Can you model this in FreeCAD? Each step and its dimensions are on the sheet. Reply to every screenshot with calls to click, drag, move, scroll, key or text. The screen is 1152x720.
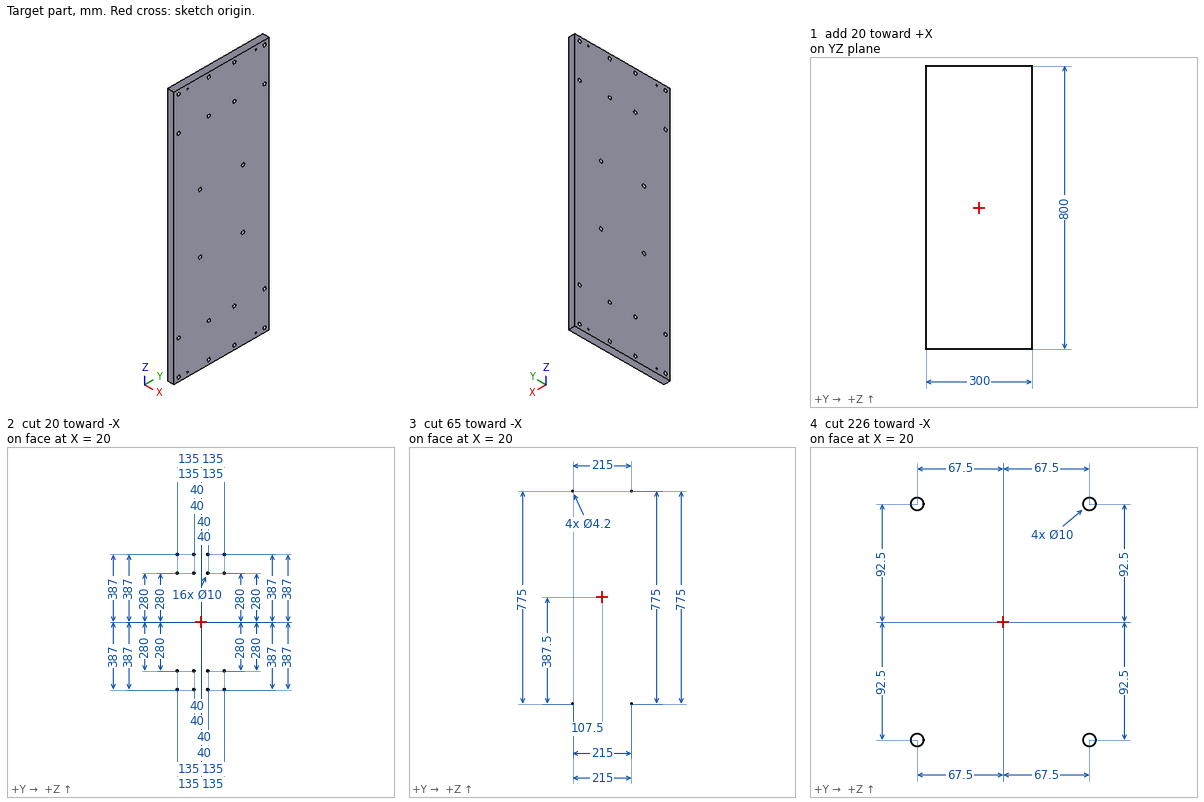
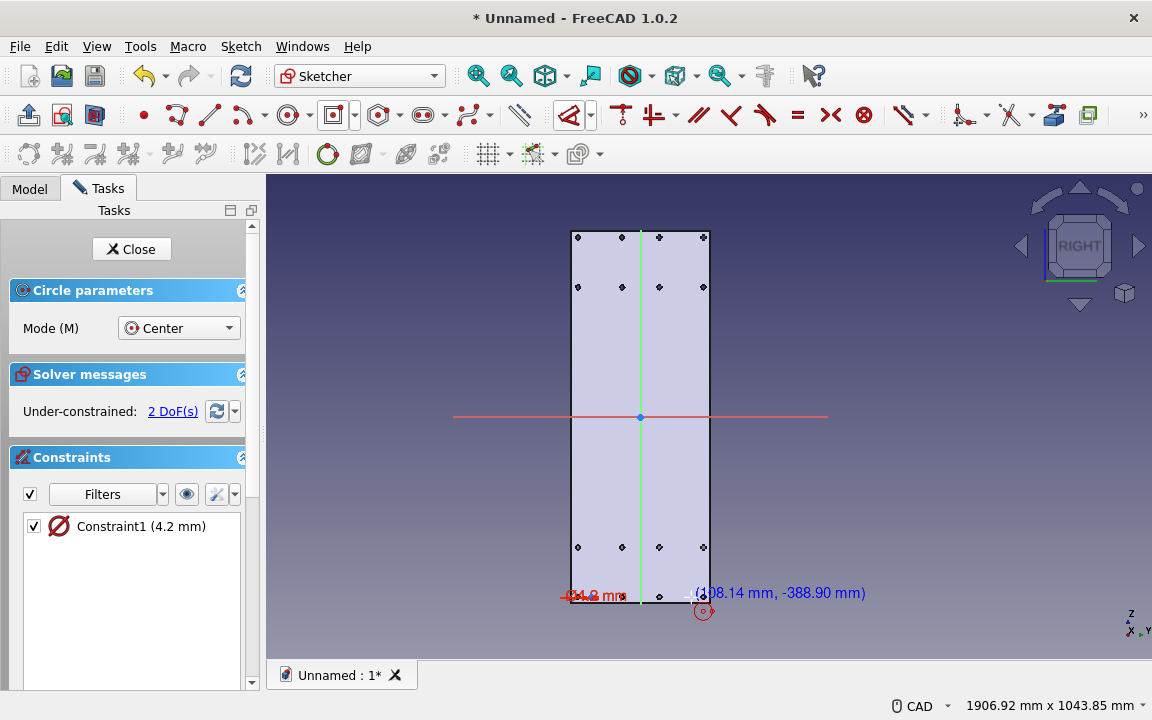
click(691, 597)
move(691, 597)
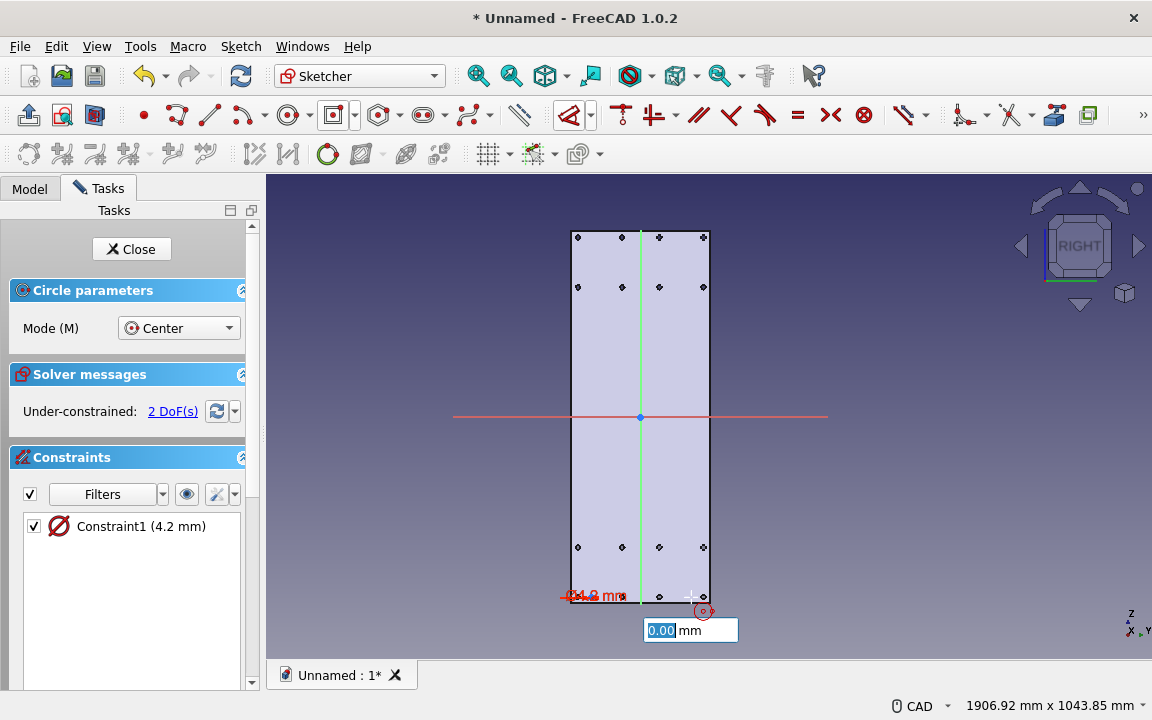
text(4.2)
key(Return)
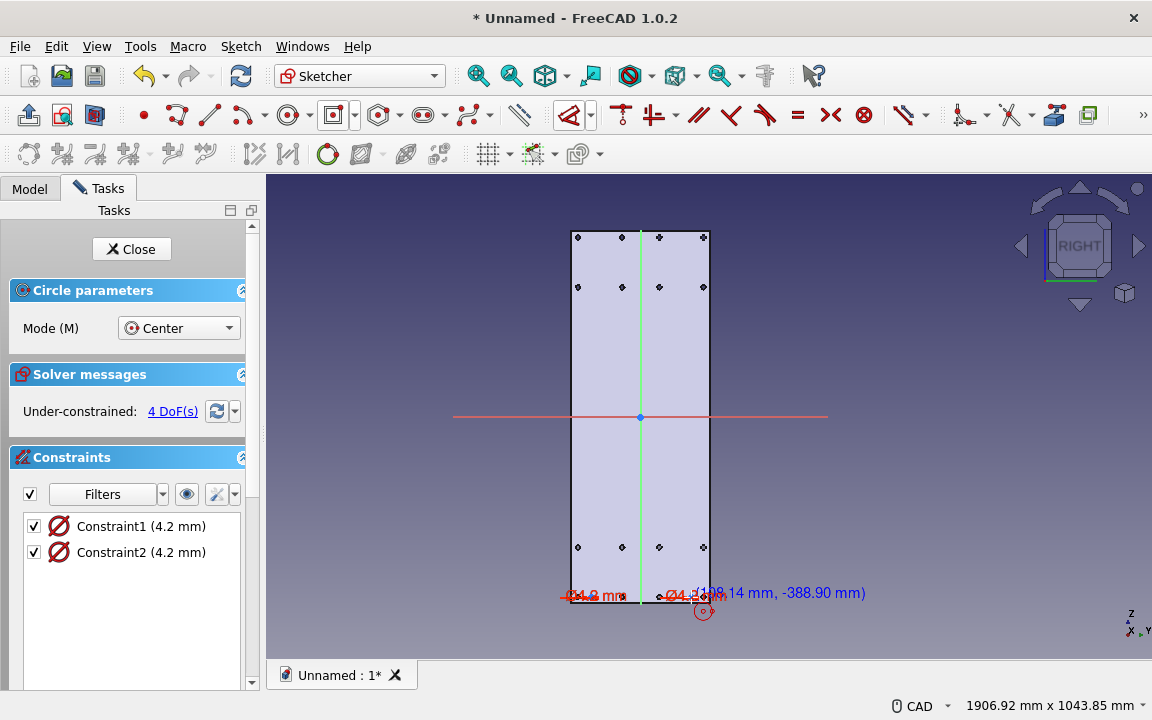
scroll(591, 237, up, 16)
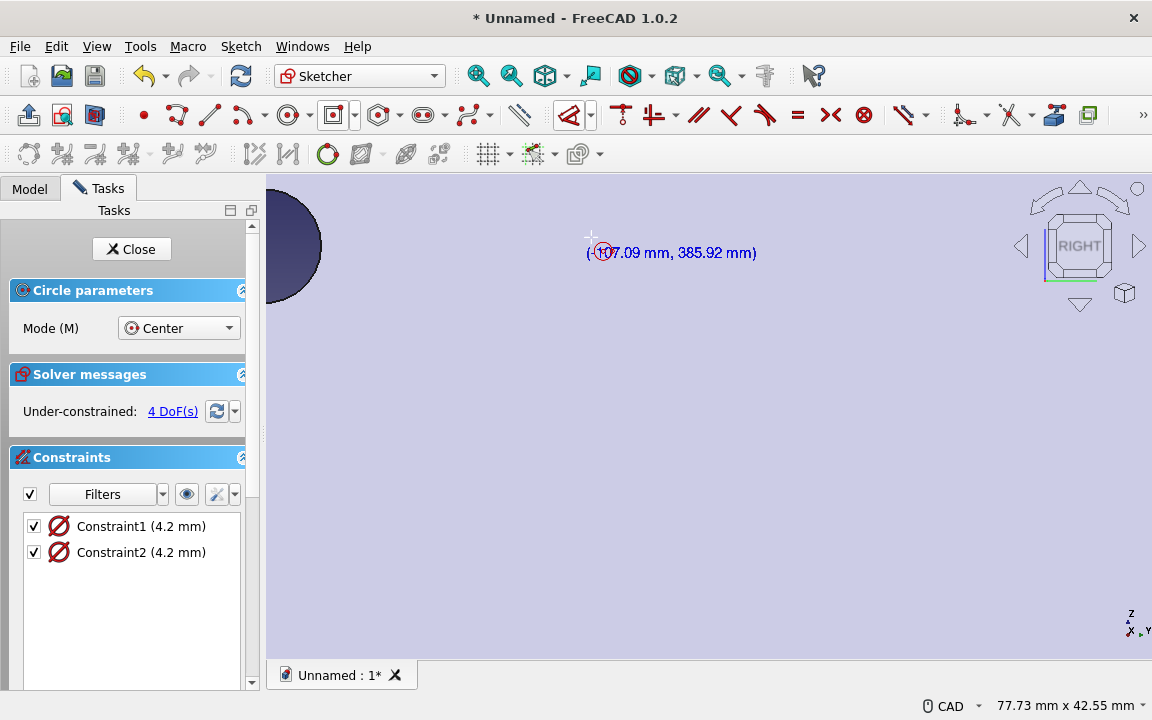
scroll(591, 236, down, 16)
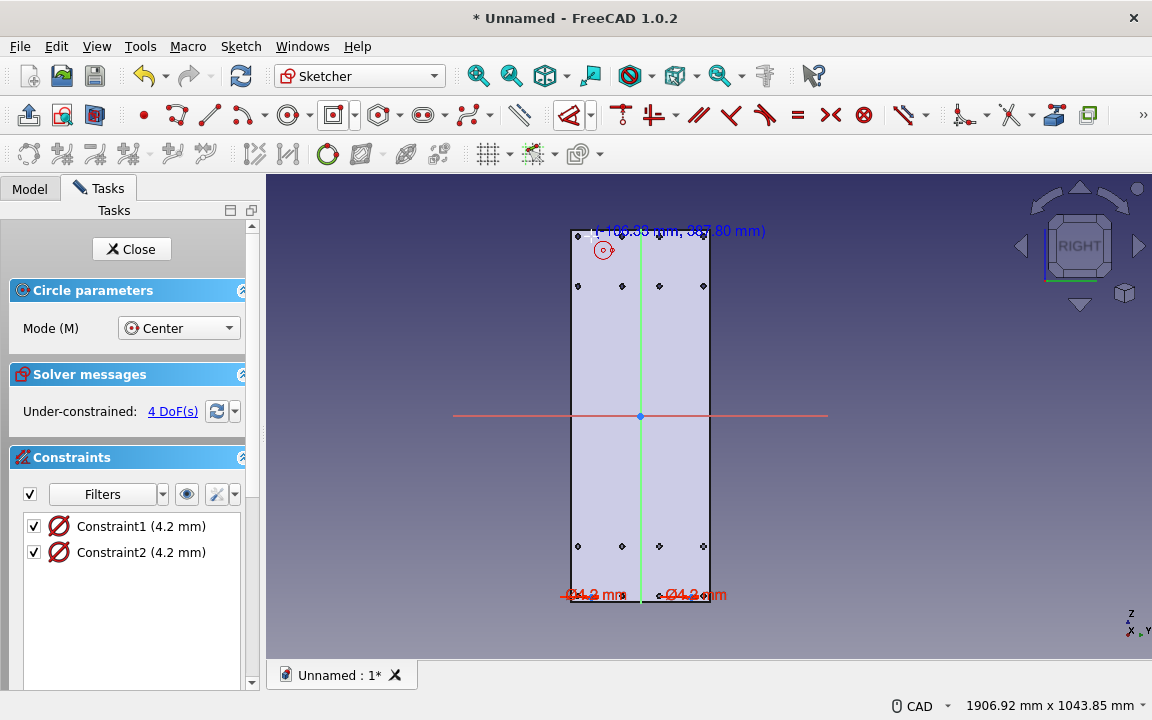
click(591, 236)
move(592, 236)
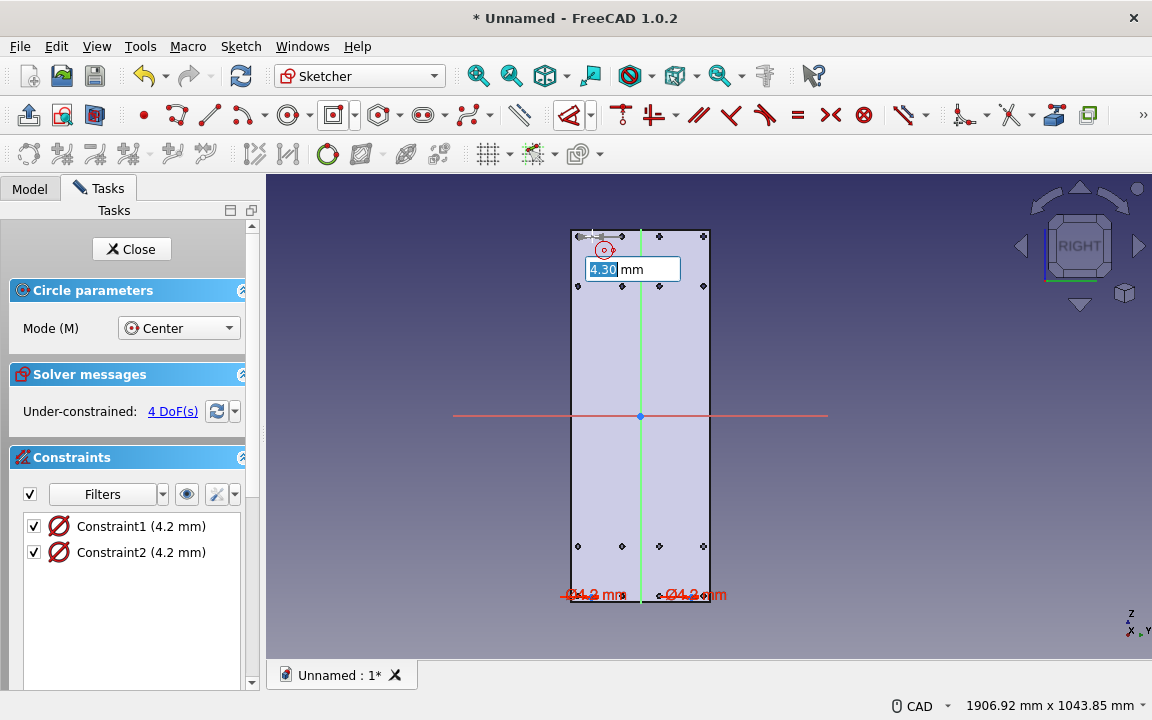
text(4.2)
key(Return)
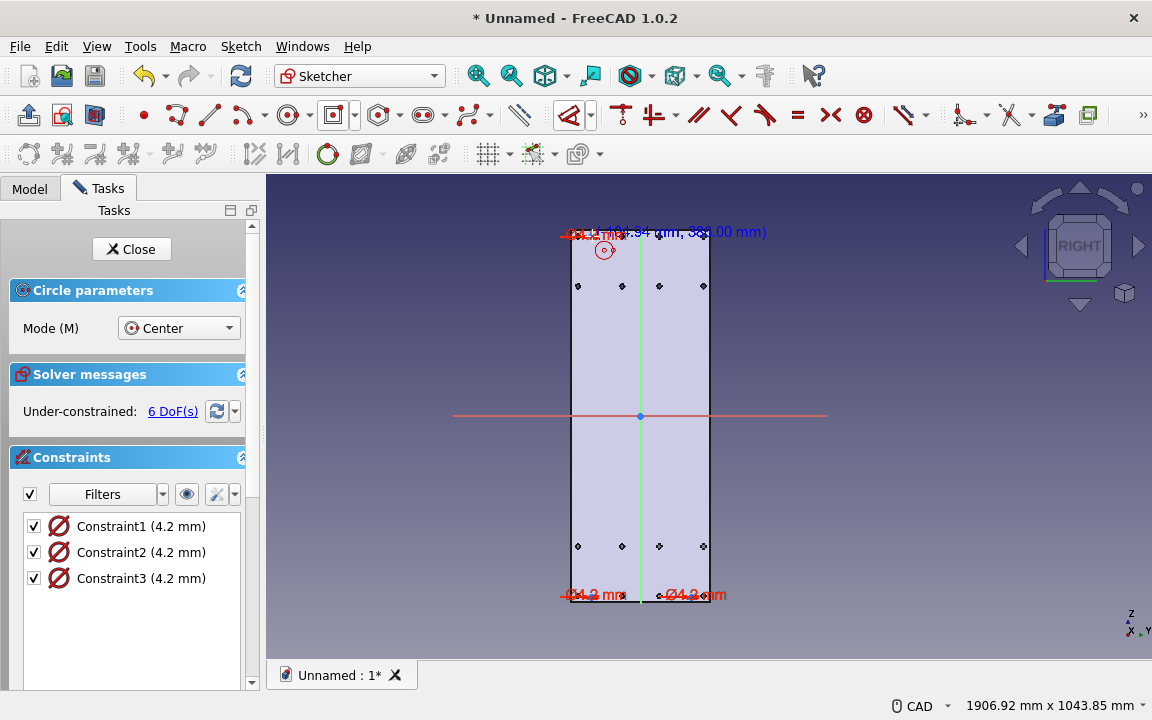
scroll(691, 236, up, 16)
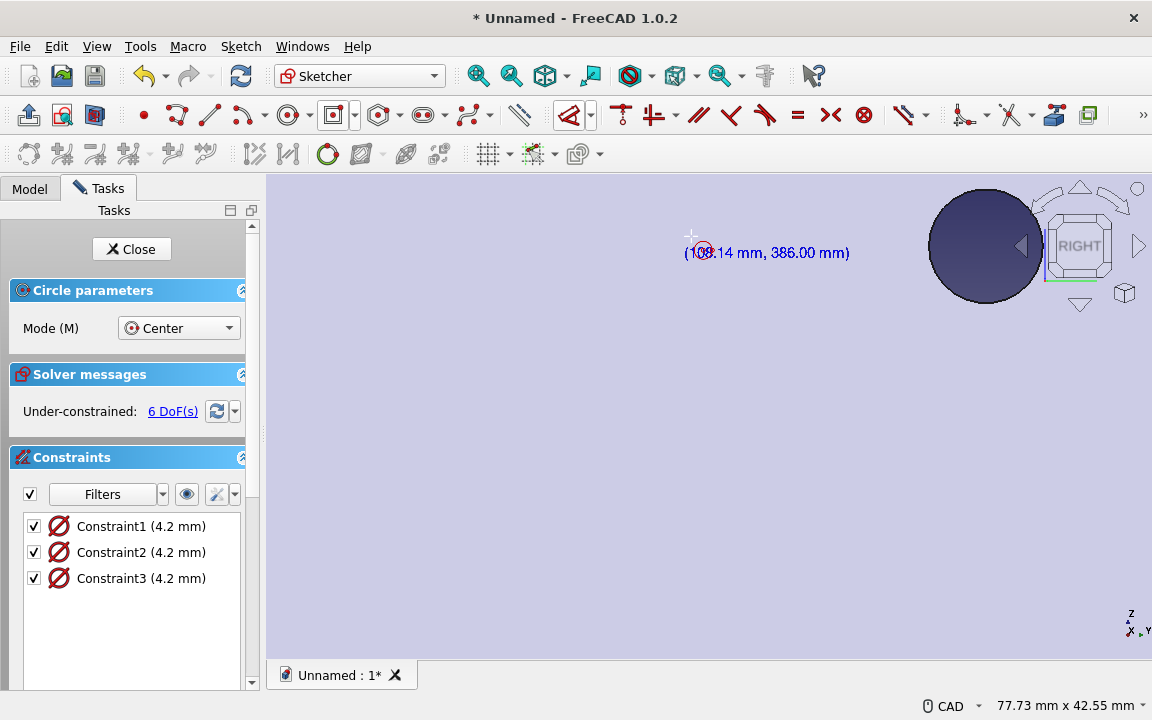
scroll(691, 236, down, 16)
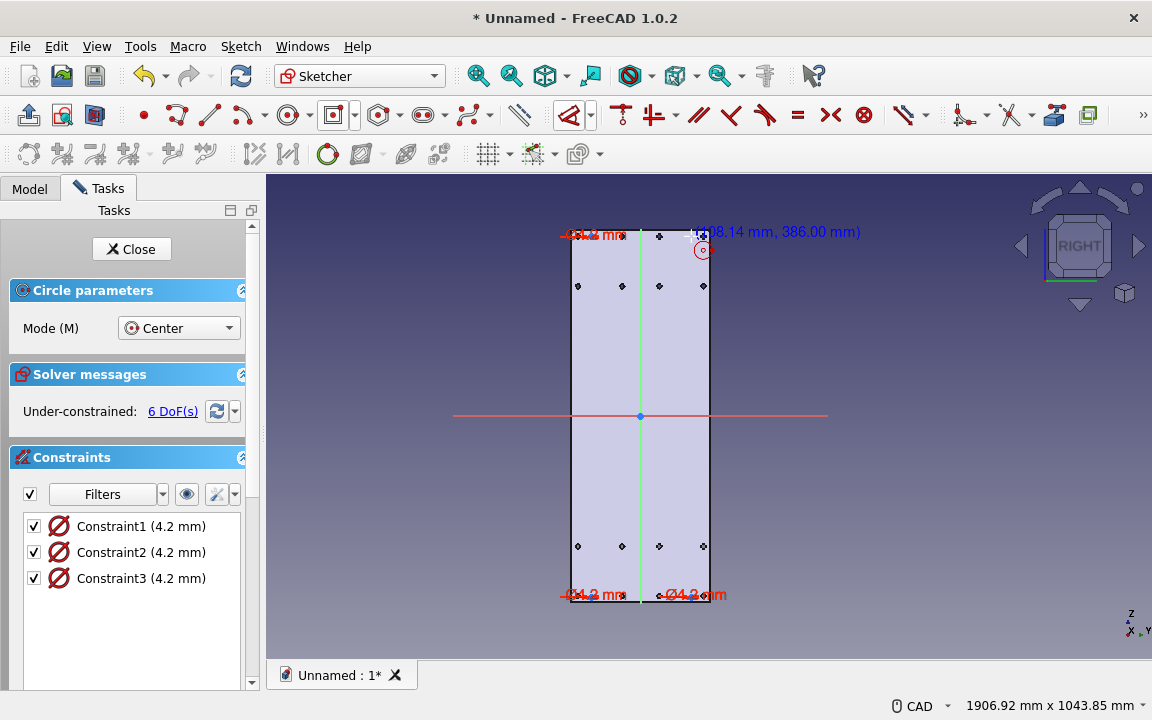
click(691, 236)
move(691, 236)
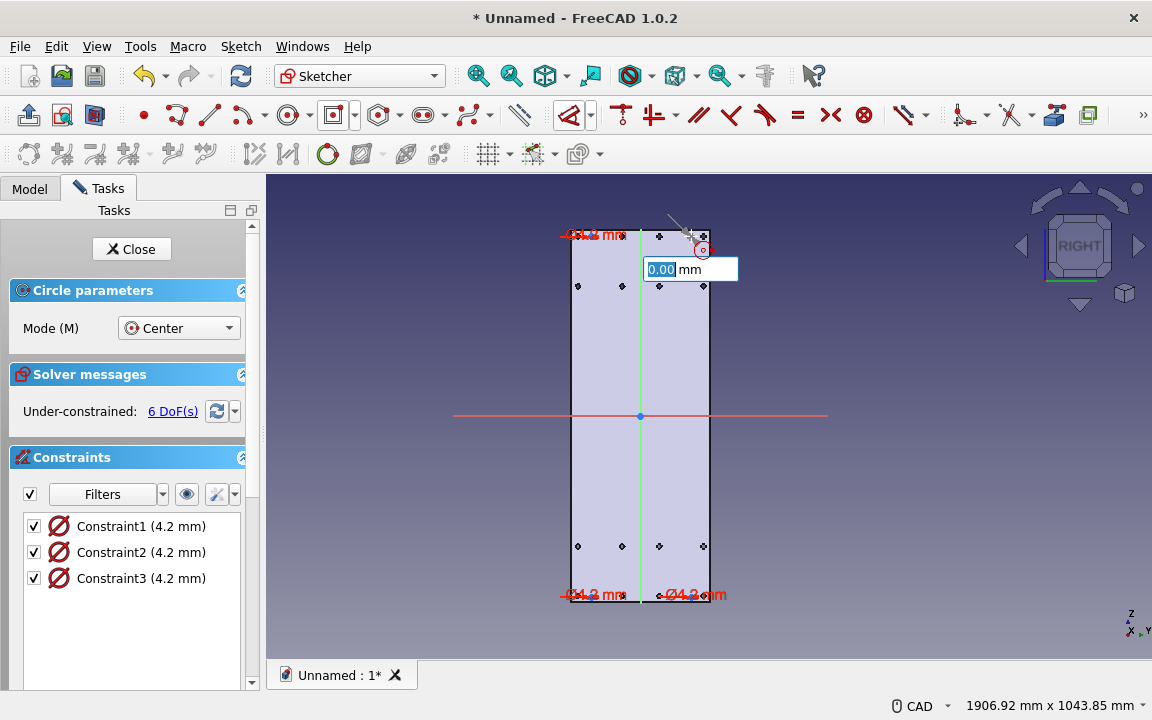
text(4.2)
key(Return)
key(Escape)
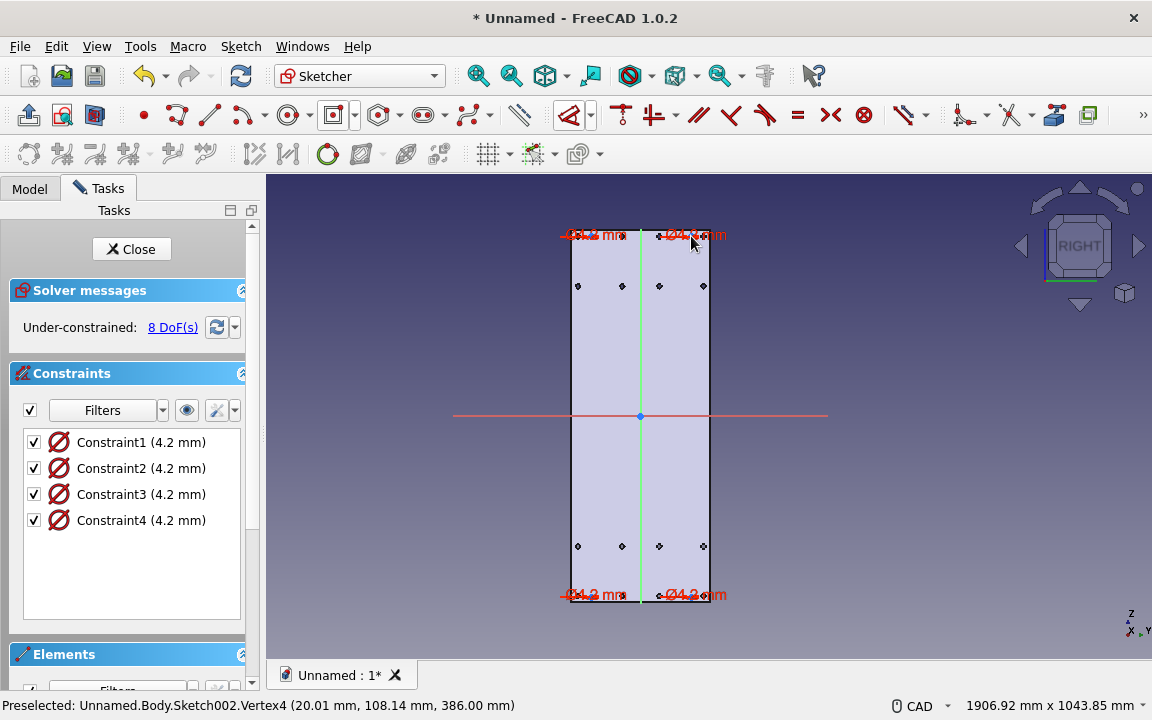
click(591, 597)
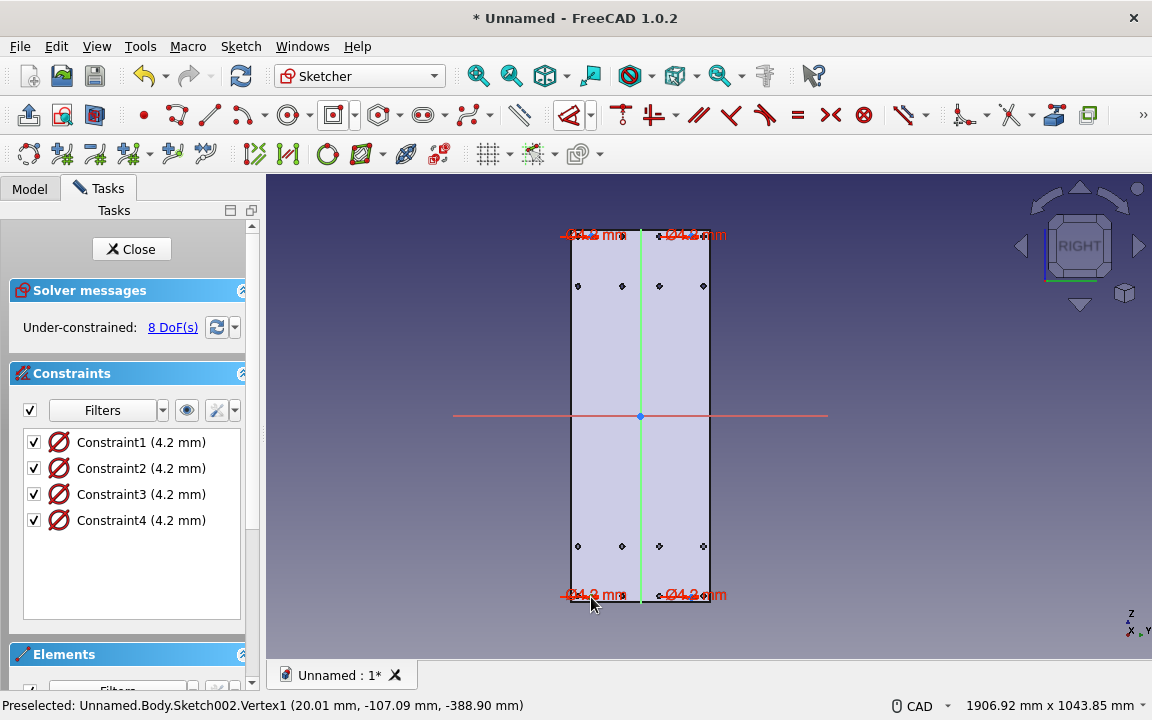
click(691, 597)